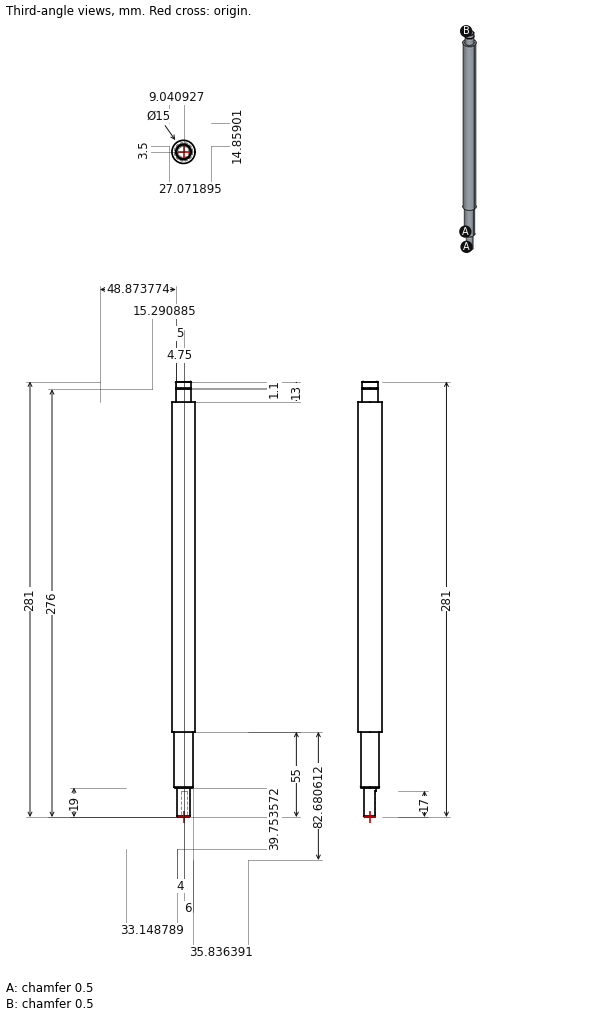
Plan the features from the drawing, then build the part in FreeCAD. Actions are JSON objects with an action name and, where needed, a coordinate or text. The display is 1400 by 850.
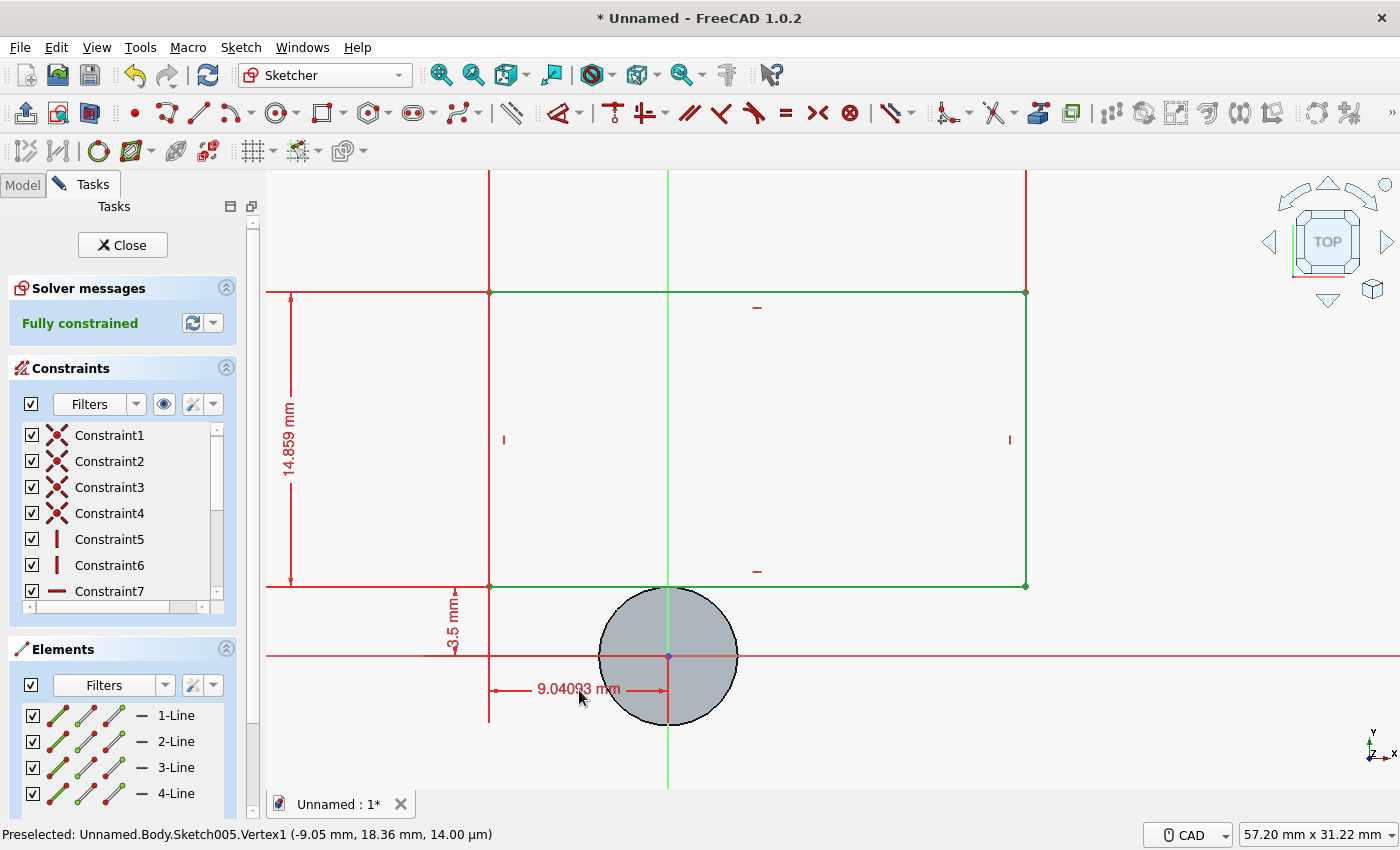
{"action": "left_click", "coordinate": [123, 245]}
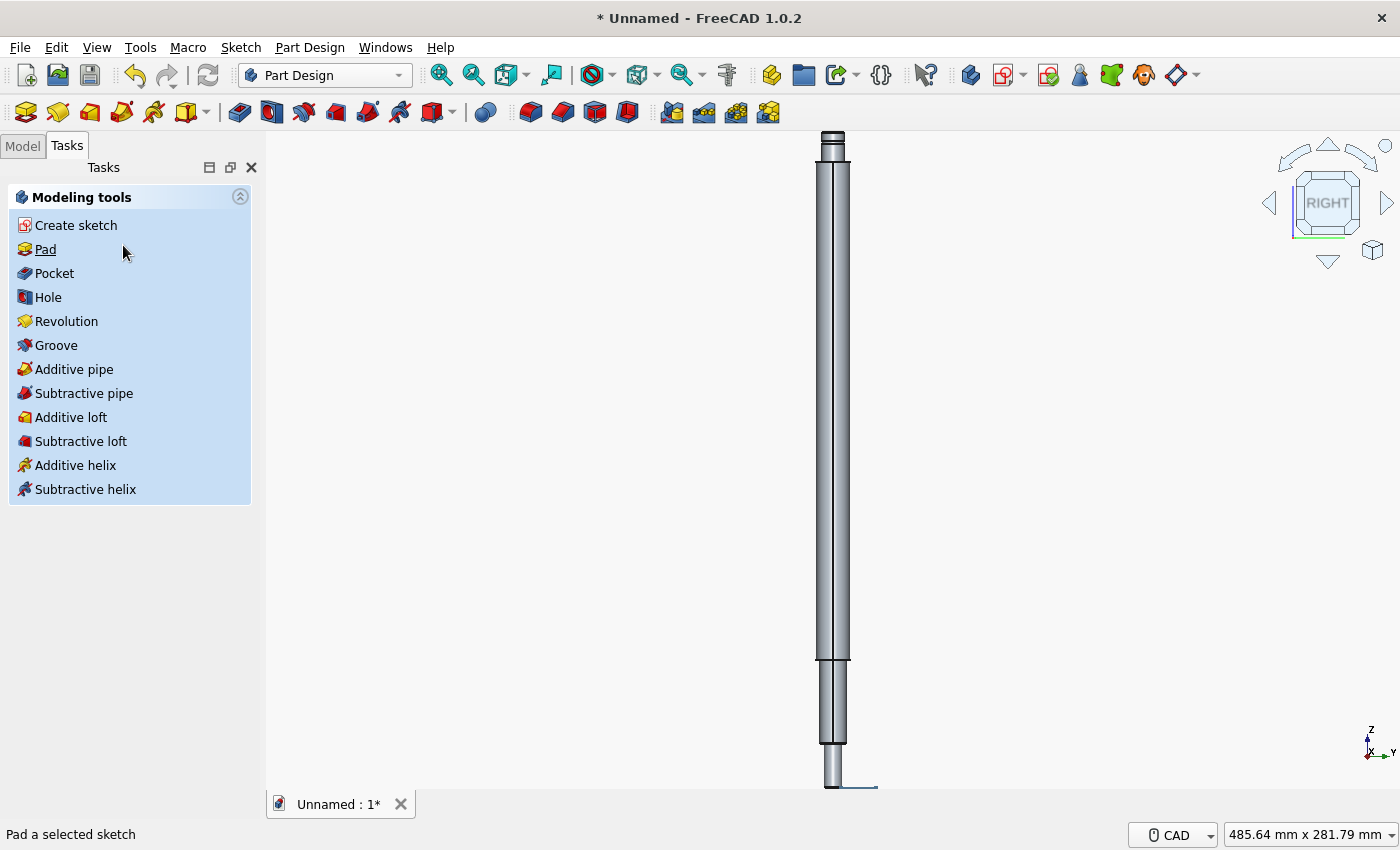
{"action": "left_click", "coordinate": [240, 112]}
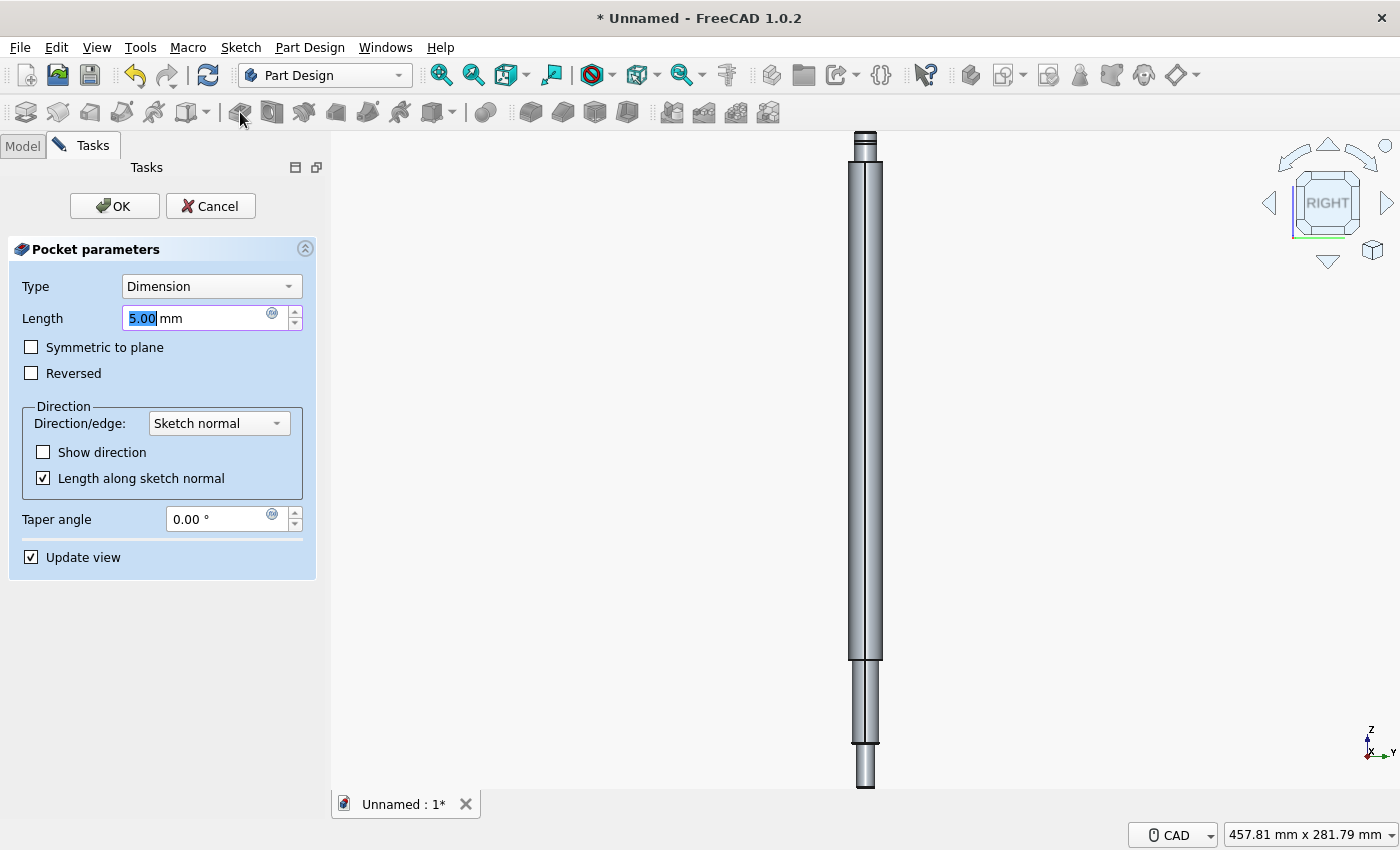
{"action": "type", "text": "17"}
{"action": "key", "text": "Tab"}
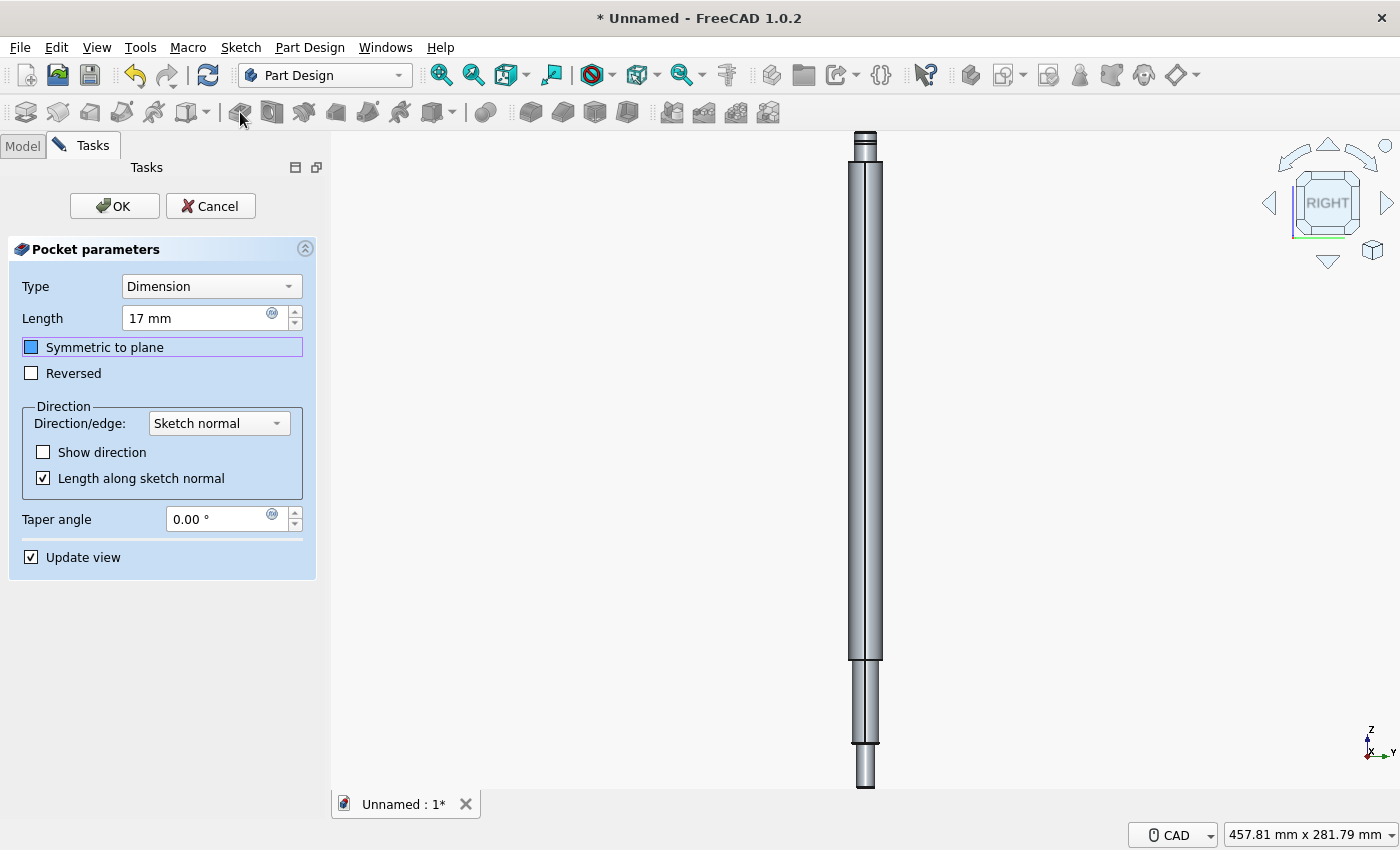
{"action": "left_click", "coordinate": [30, 373]}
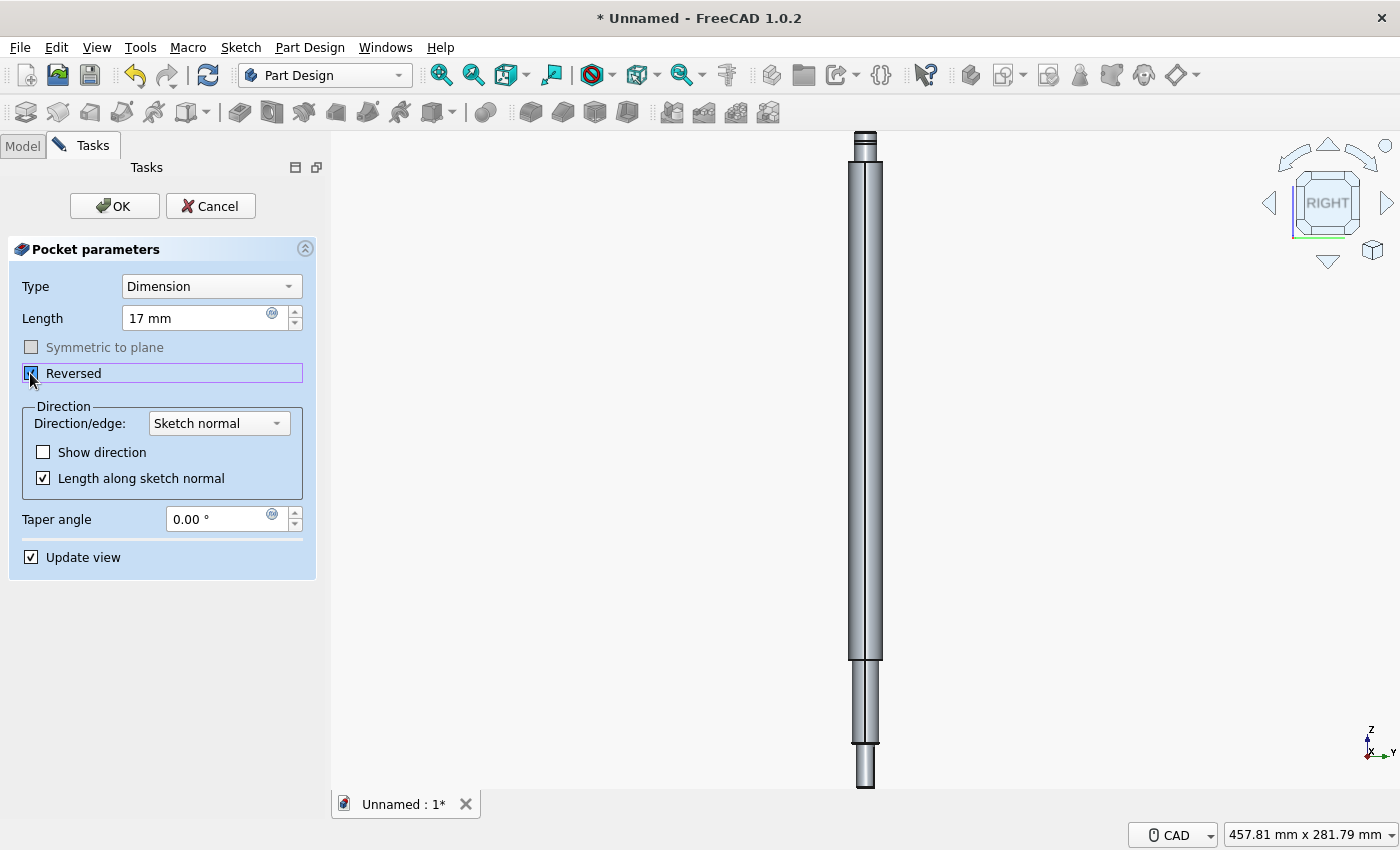
{"action": "left_click", "coordinate": [115, 206]}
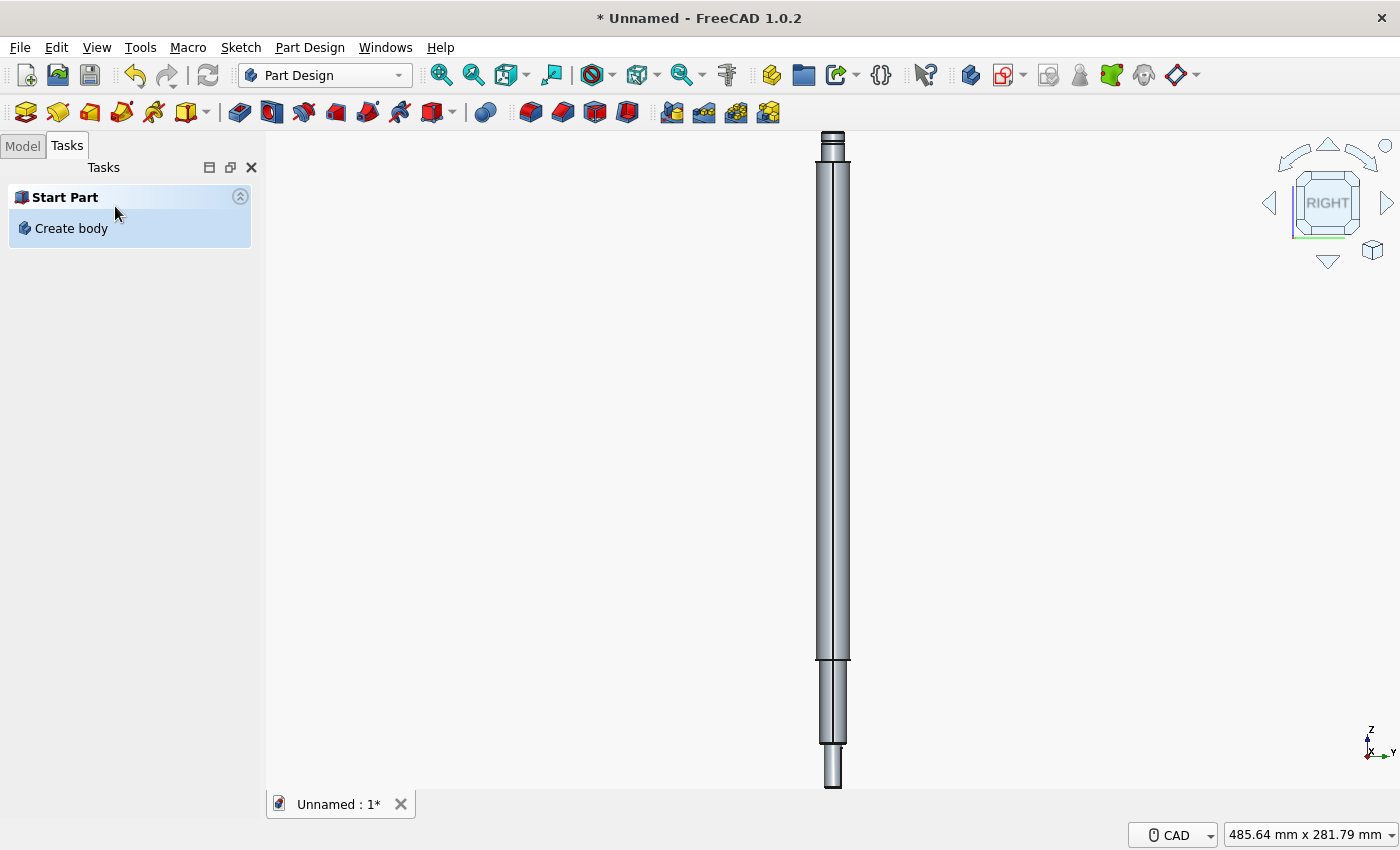
{"action": "key", "text": "0"}